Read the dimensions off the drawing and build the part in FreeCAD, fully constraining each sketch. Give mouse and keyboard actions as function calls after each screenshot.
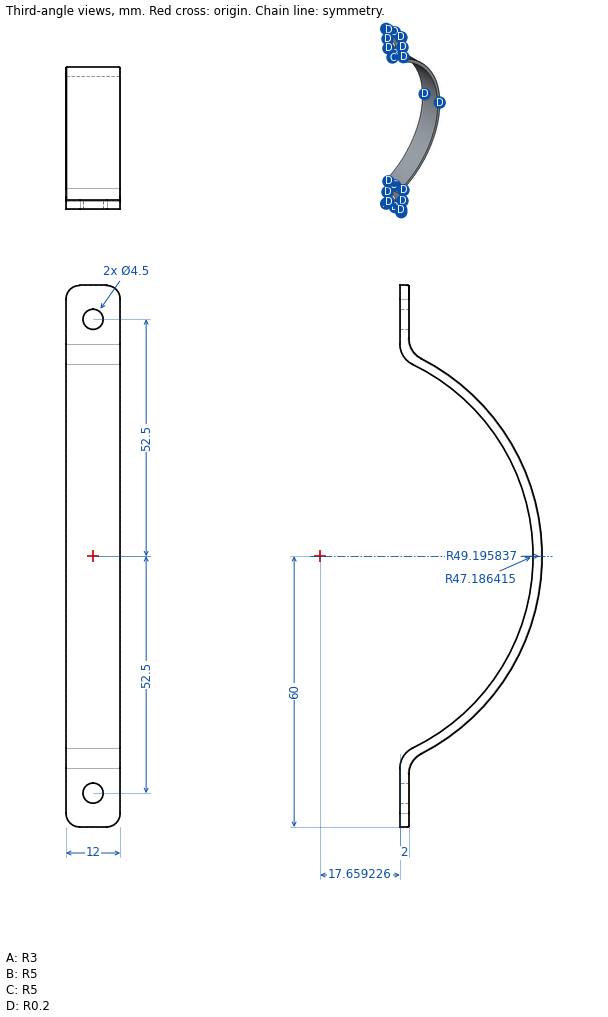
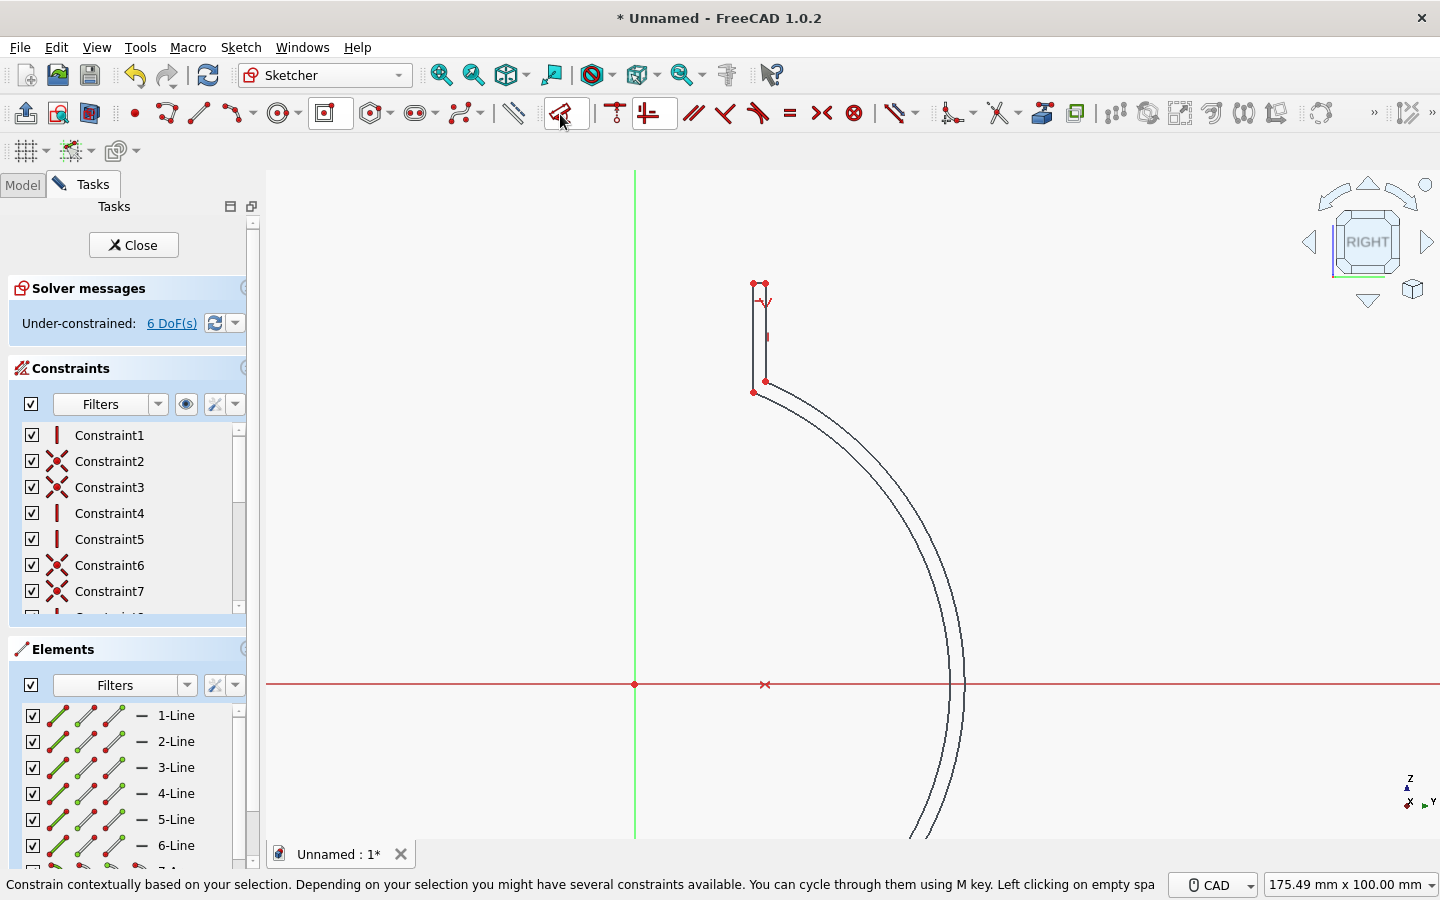
click(930, 537)
click(959, 523)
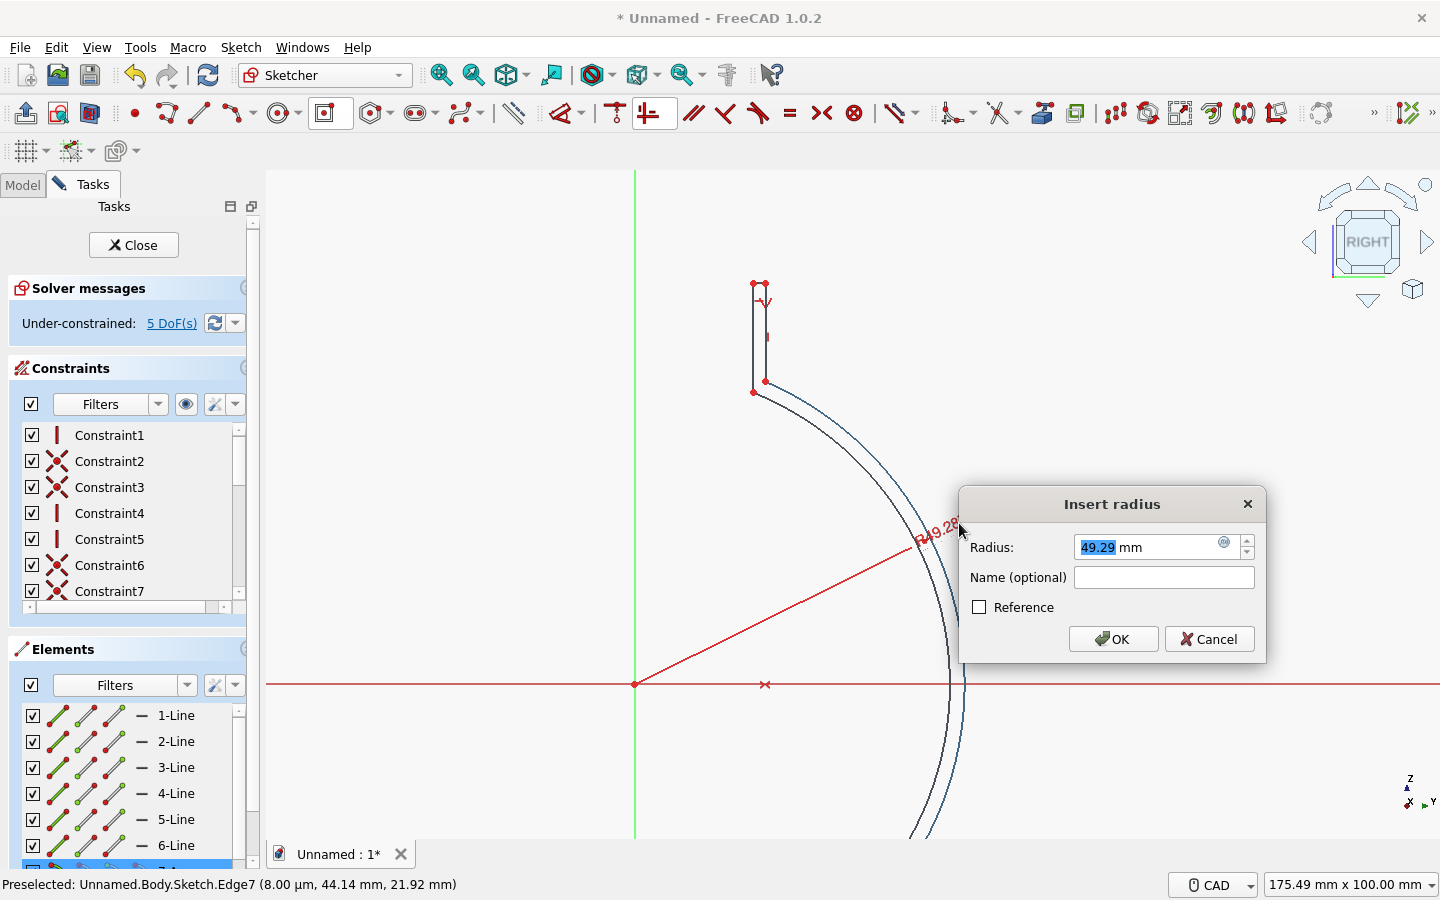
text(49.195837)
key(Return)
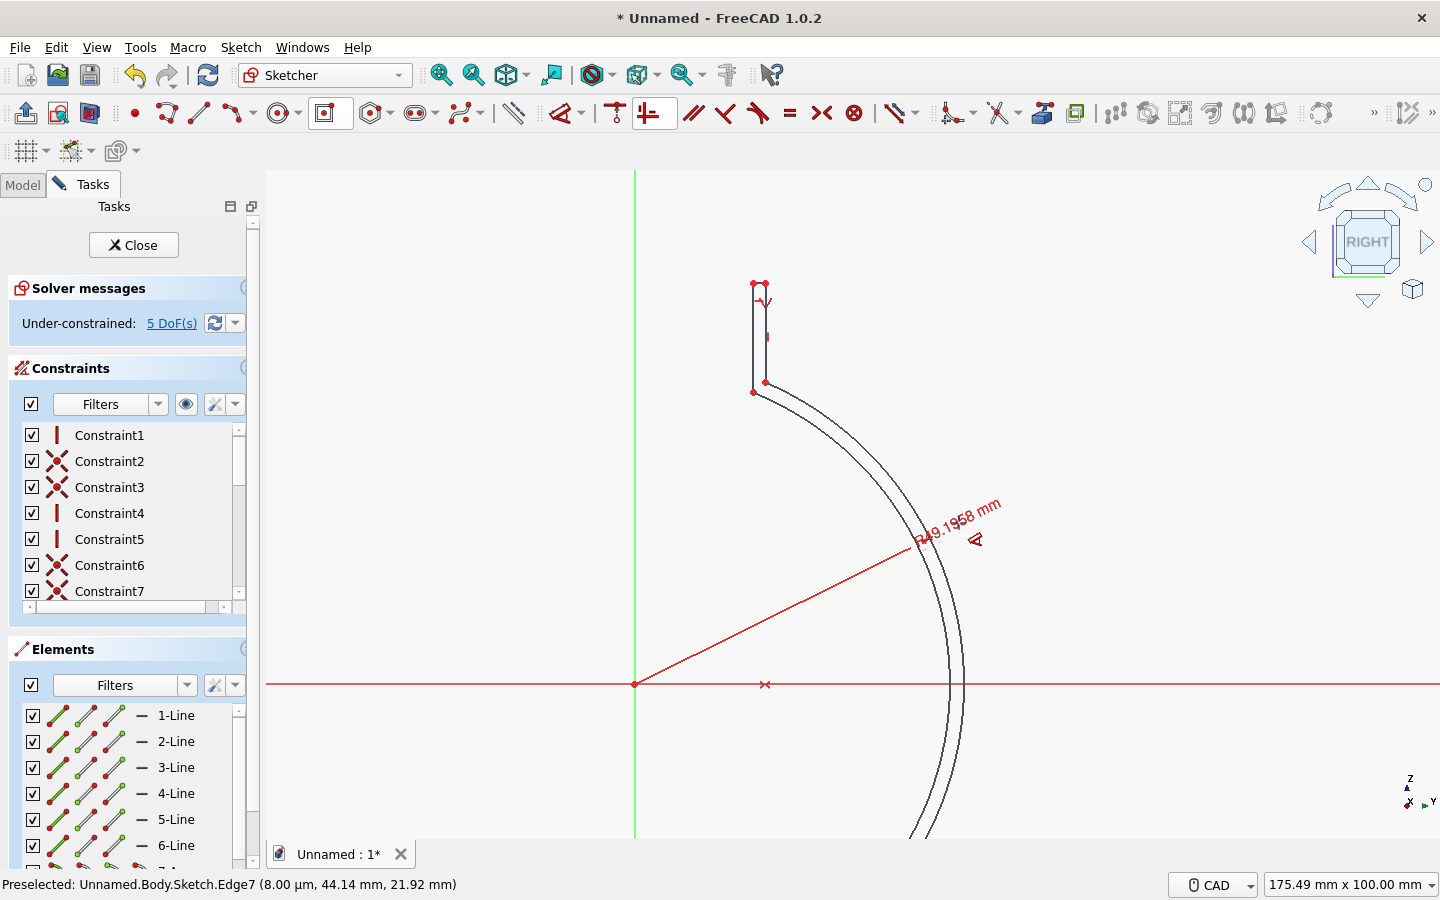
click(915, 541)
click(830, 398)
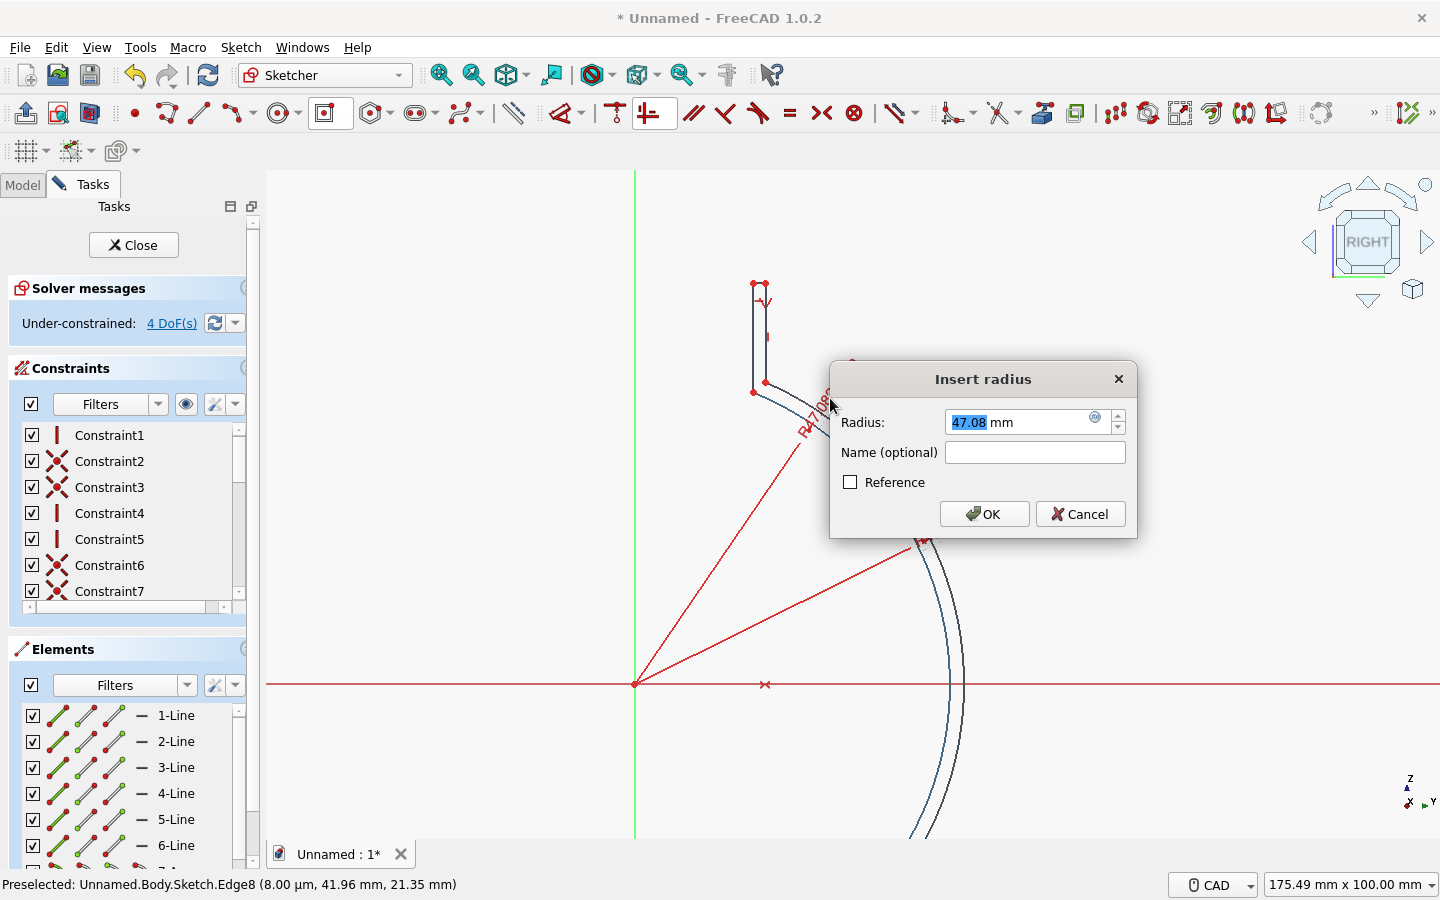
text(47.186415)
key(Return)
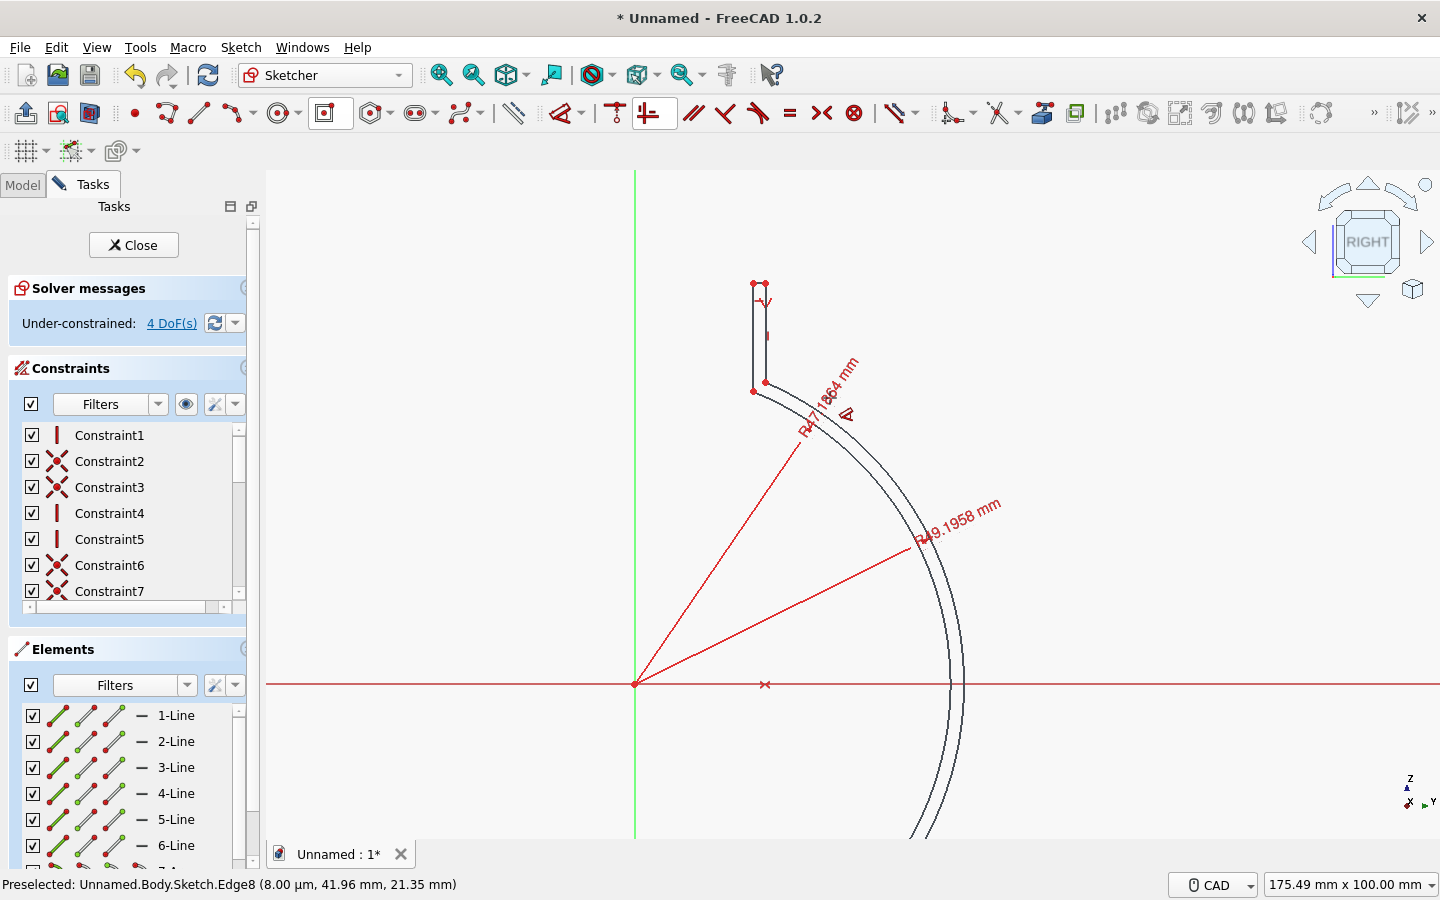
scroll(766, 286, down, 3)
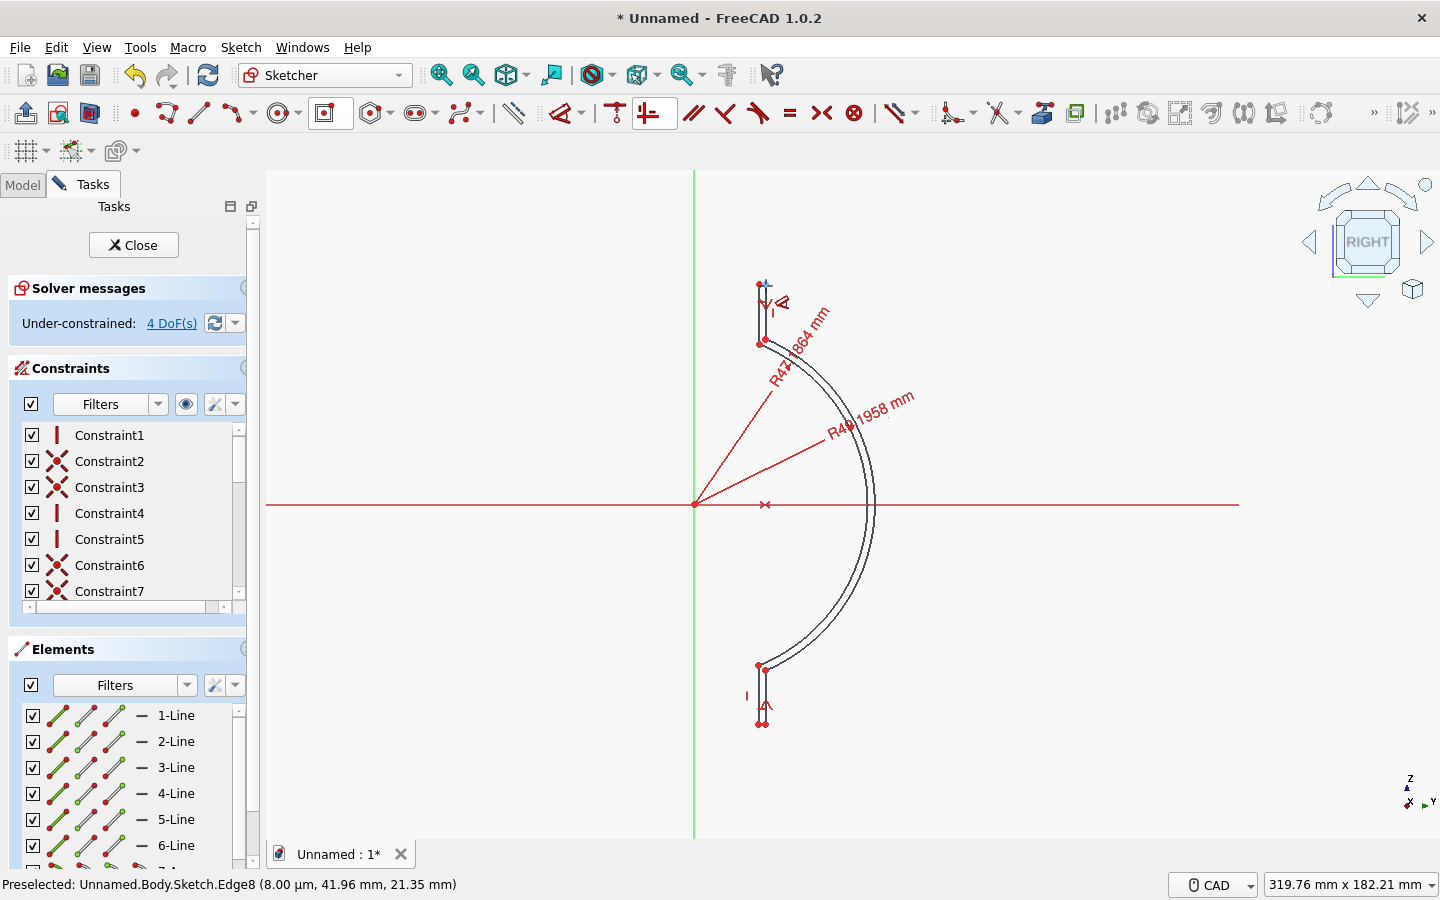
scroll(762, 725, up, 9)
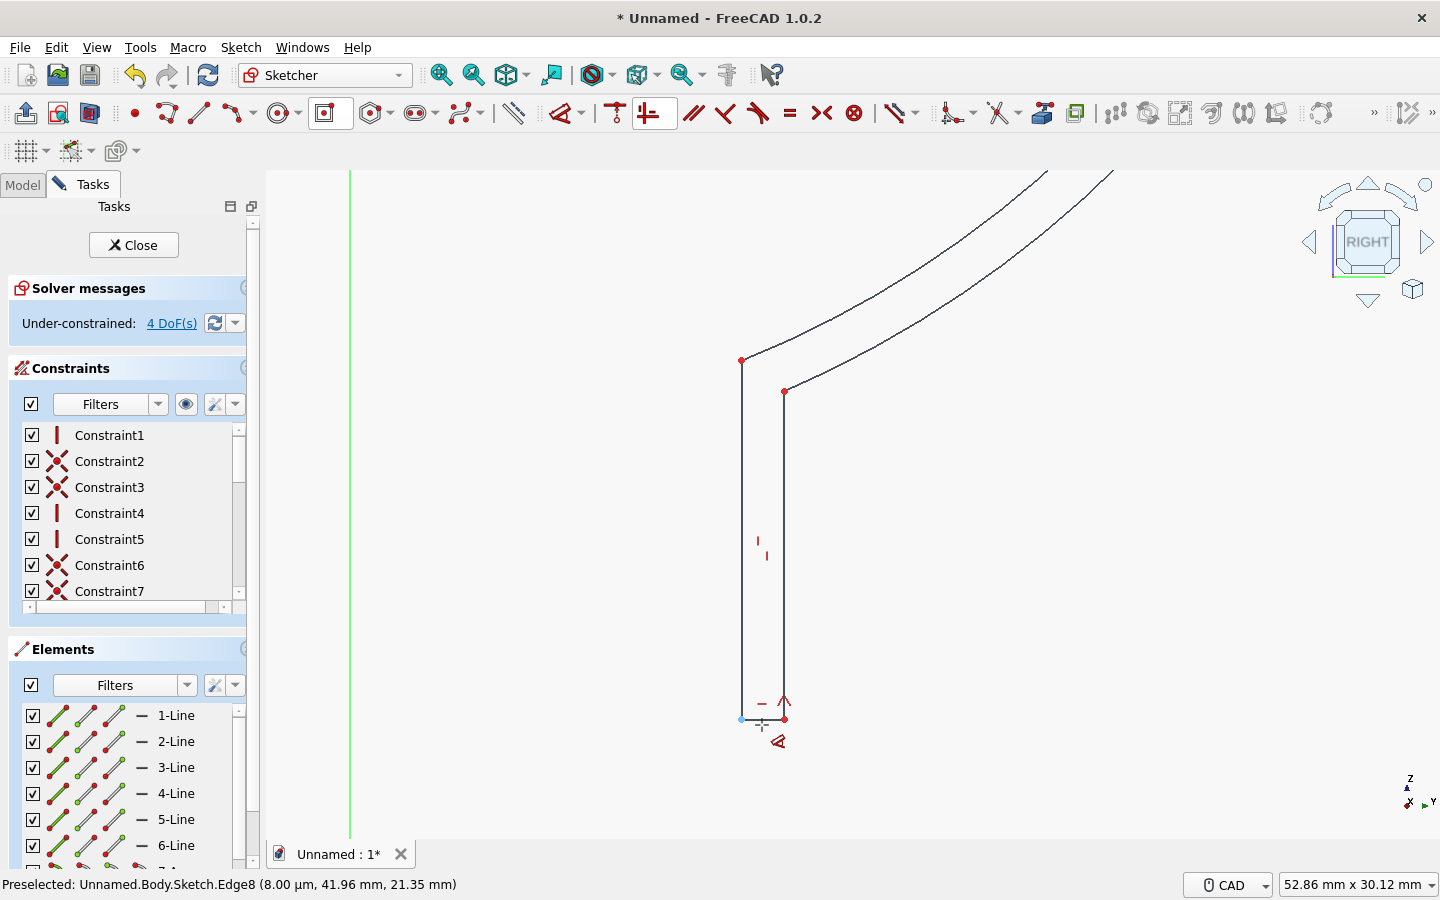
click(763, 720)
click(763, 754)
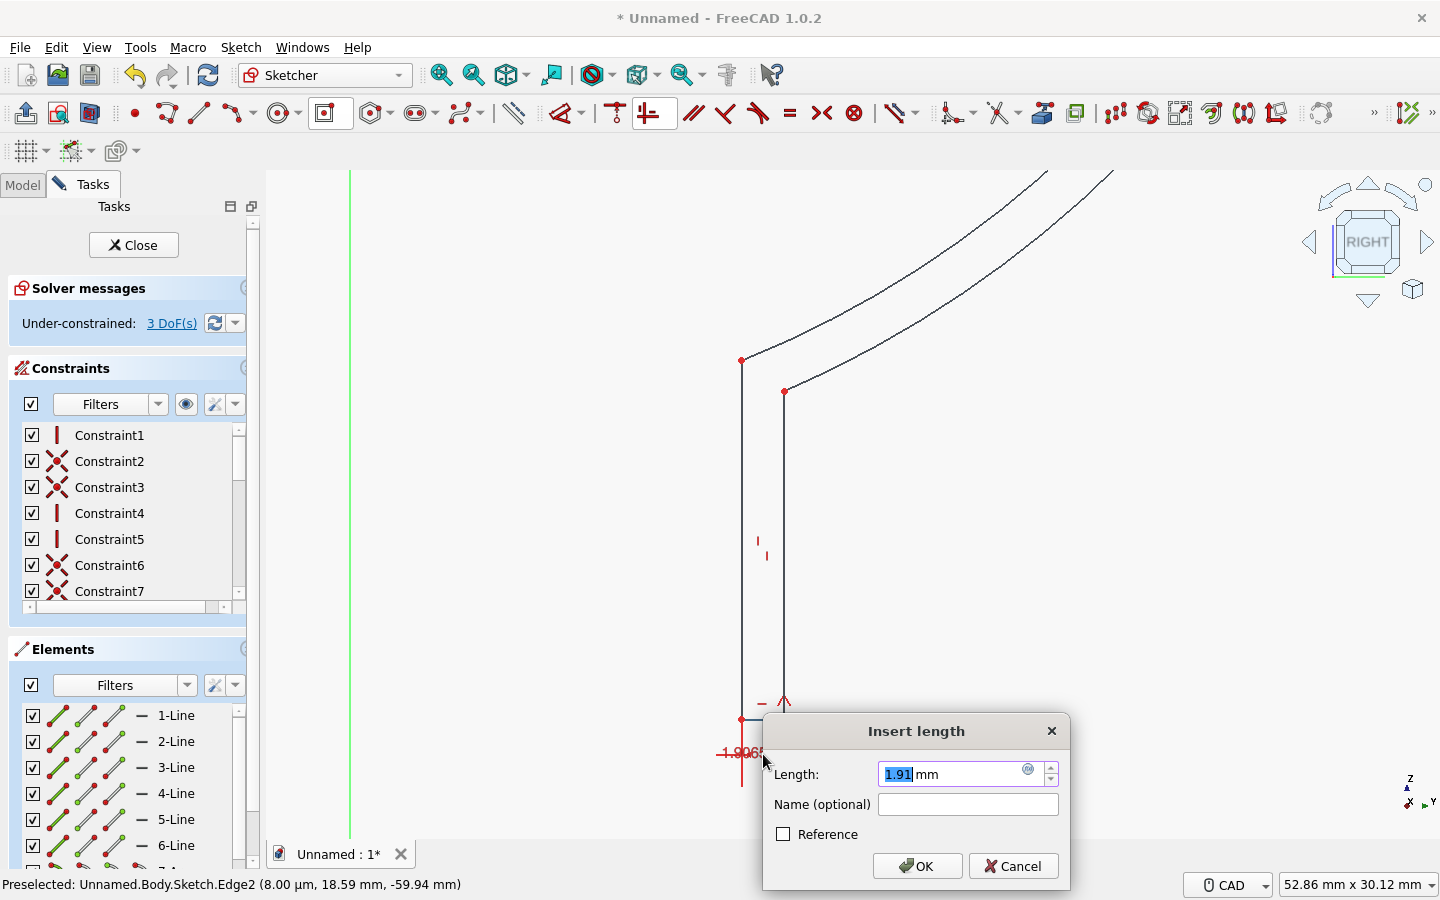
text(2)
key(Return)